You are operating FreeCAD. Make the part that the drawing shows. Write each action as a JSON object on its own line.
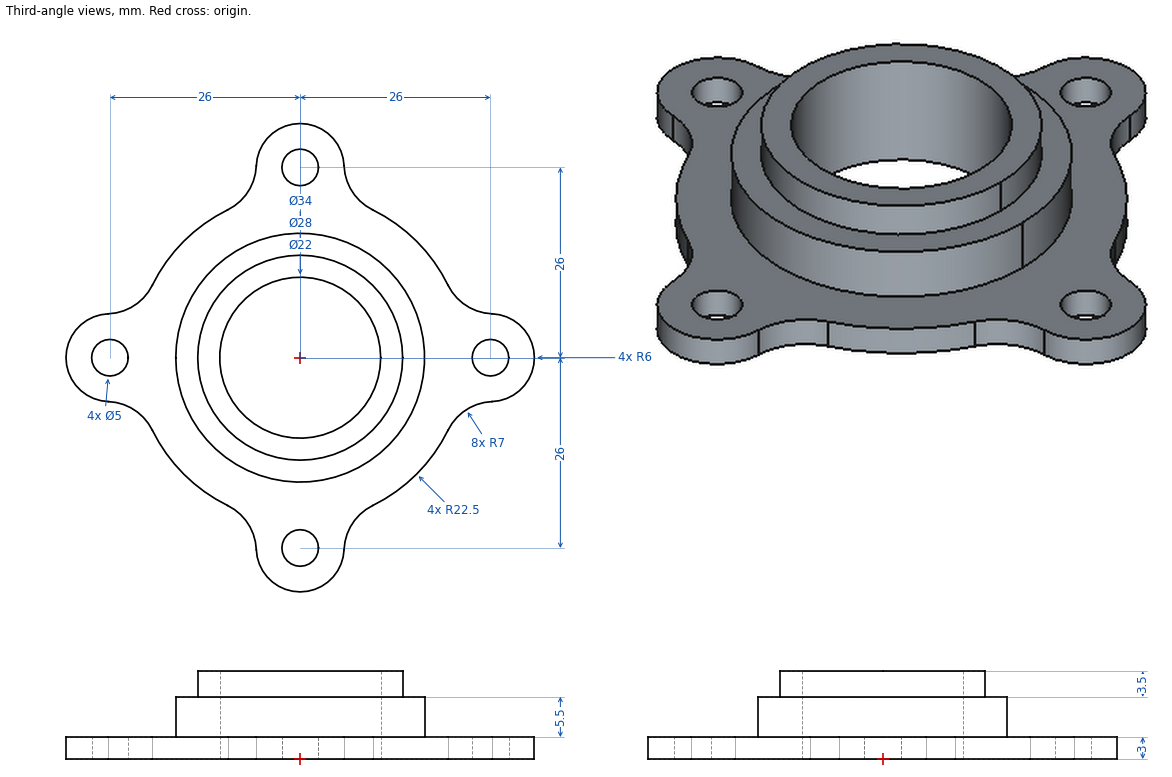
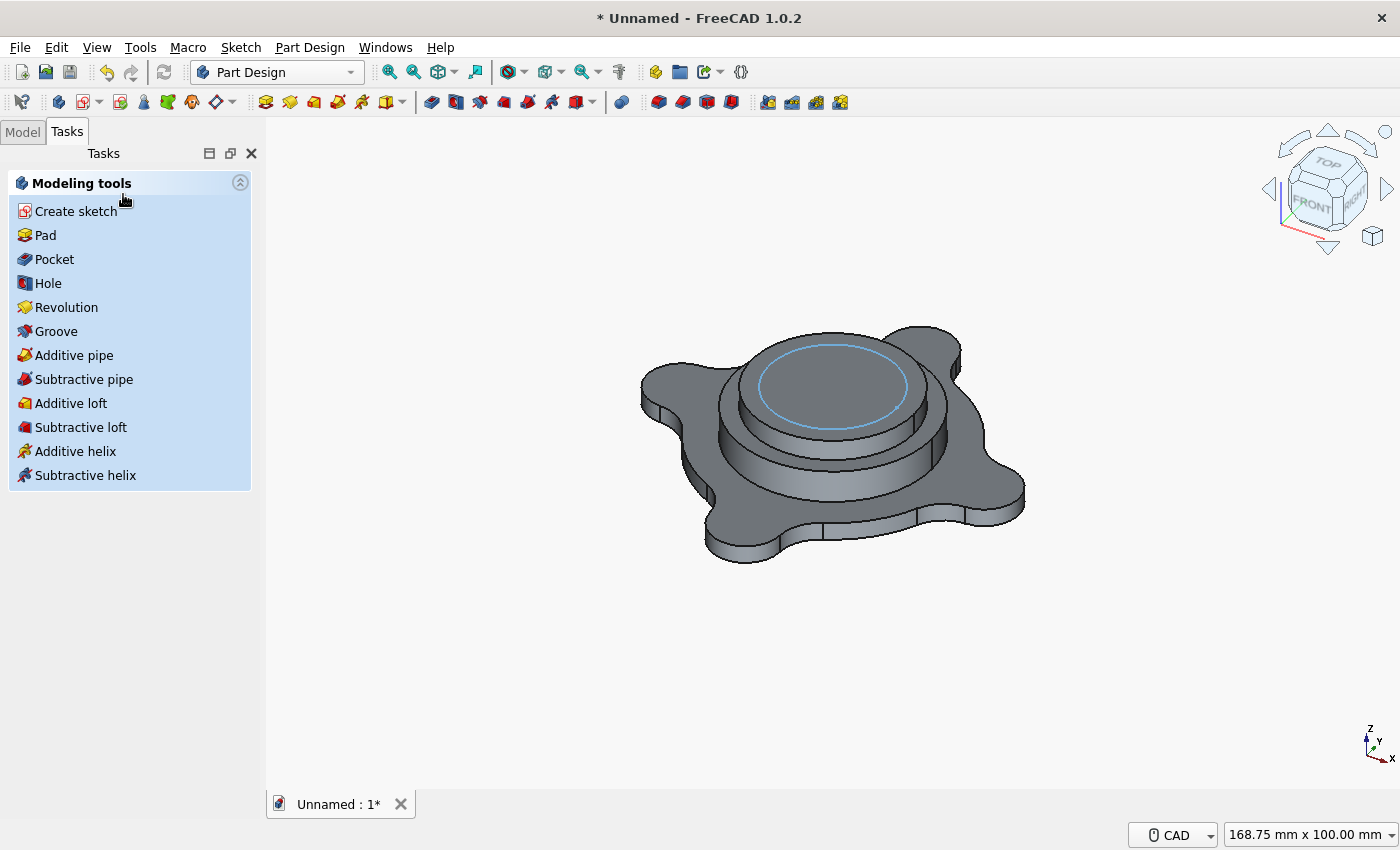
{"action": "left_click", "coordinate": [432, 102]}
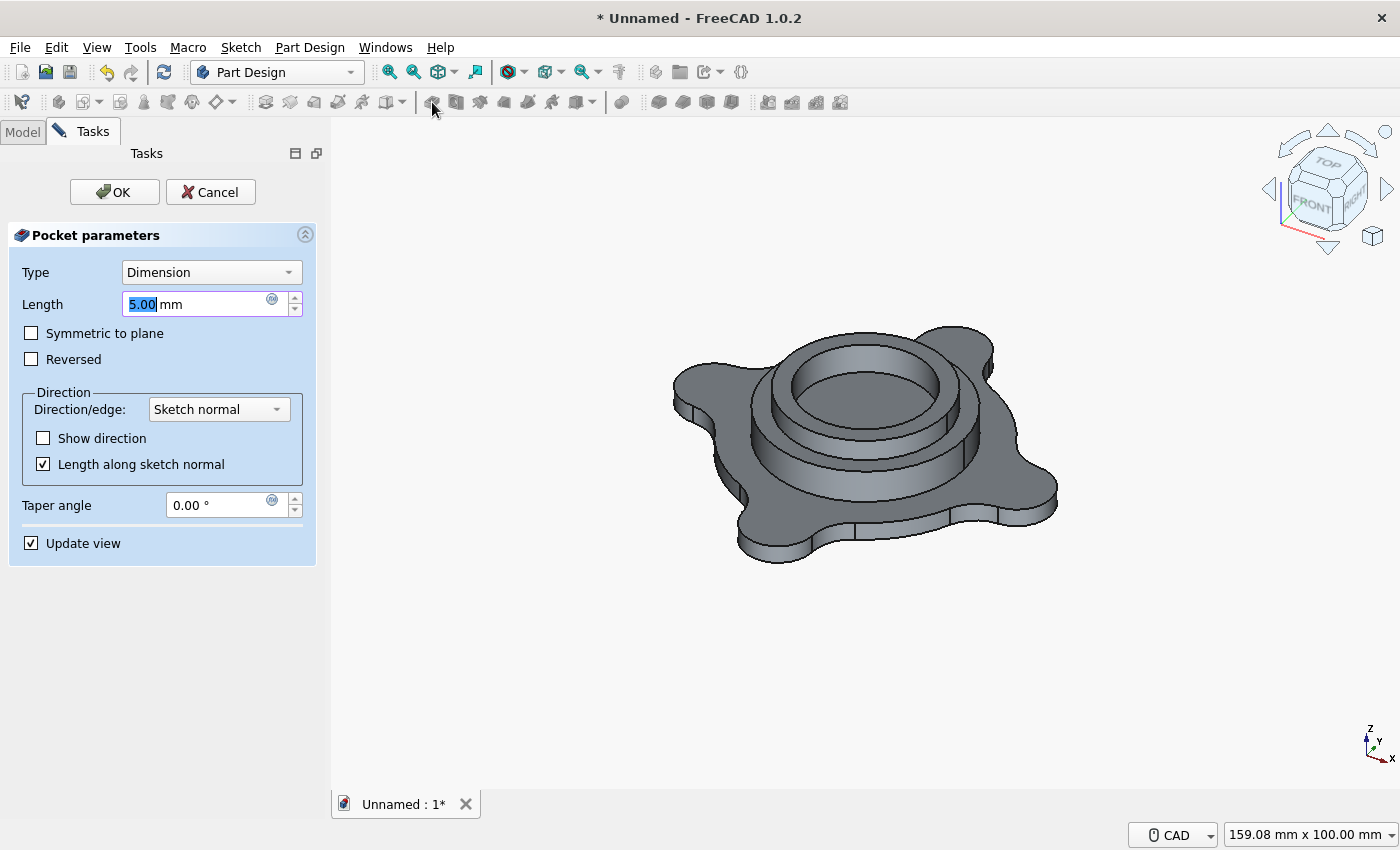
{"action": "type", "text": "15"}
{"action": "key", "text": "Tab"}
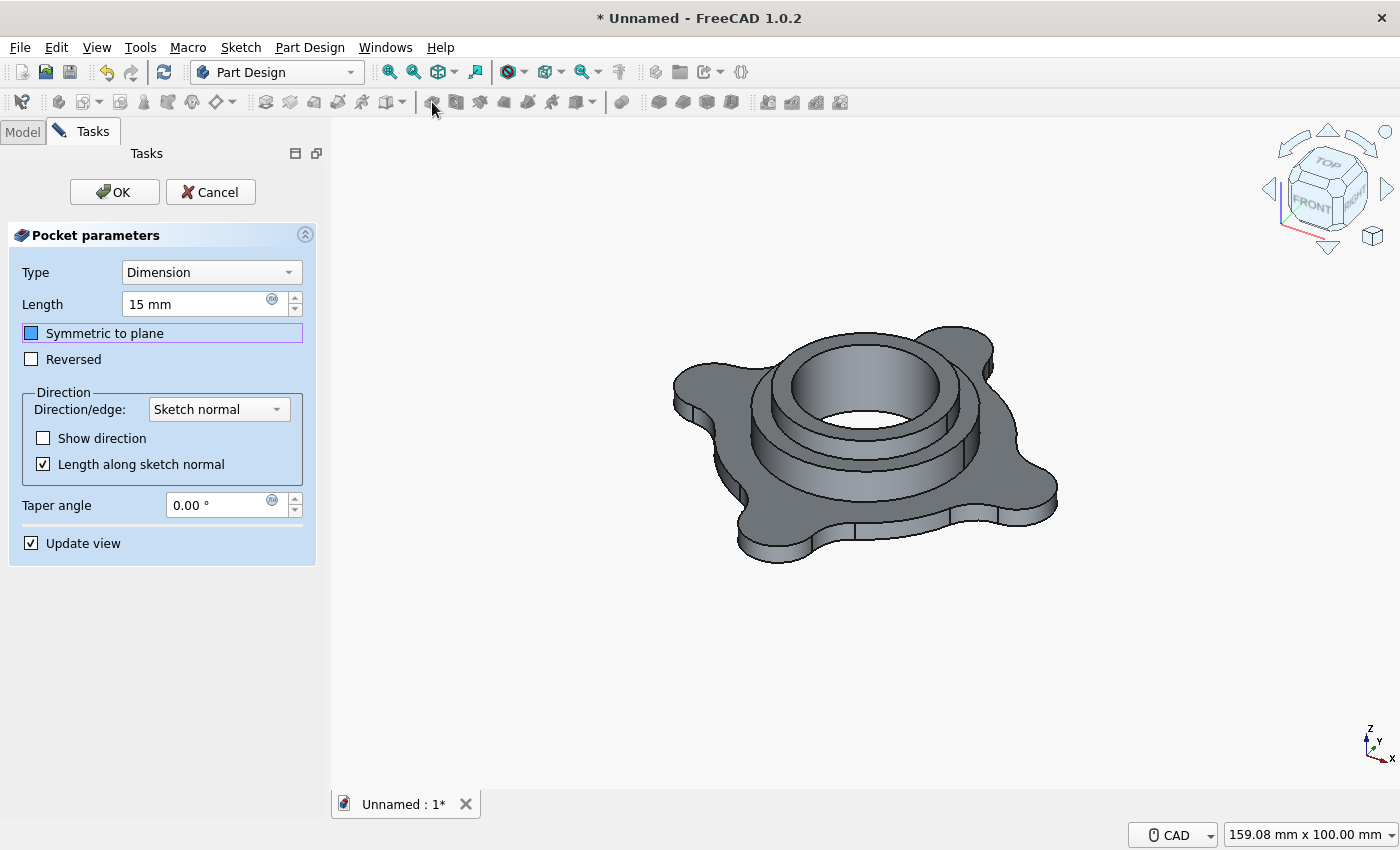
{"action": "left_click", "coordinate": [115, 192]}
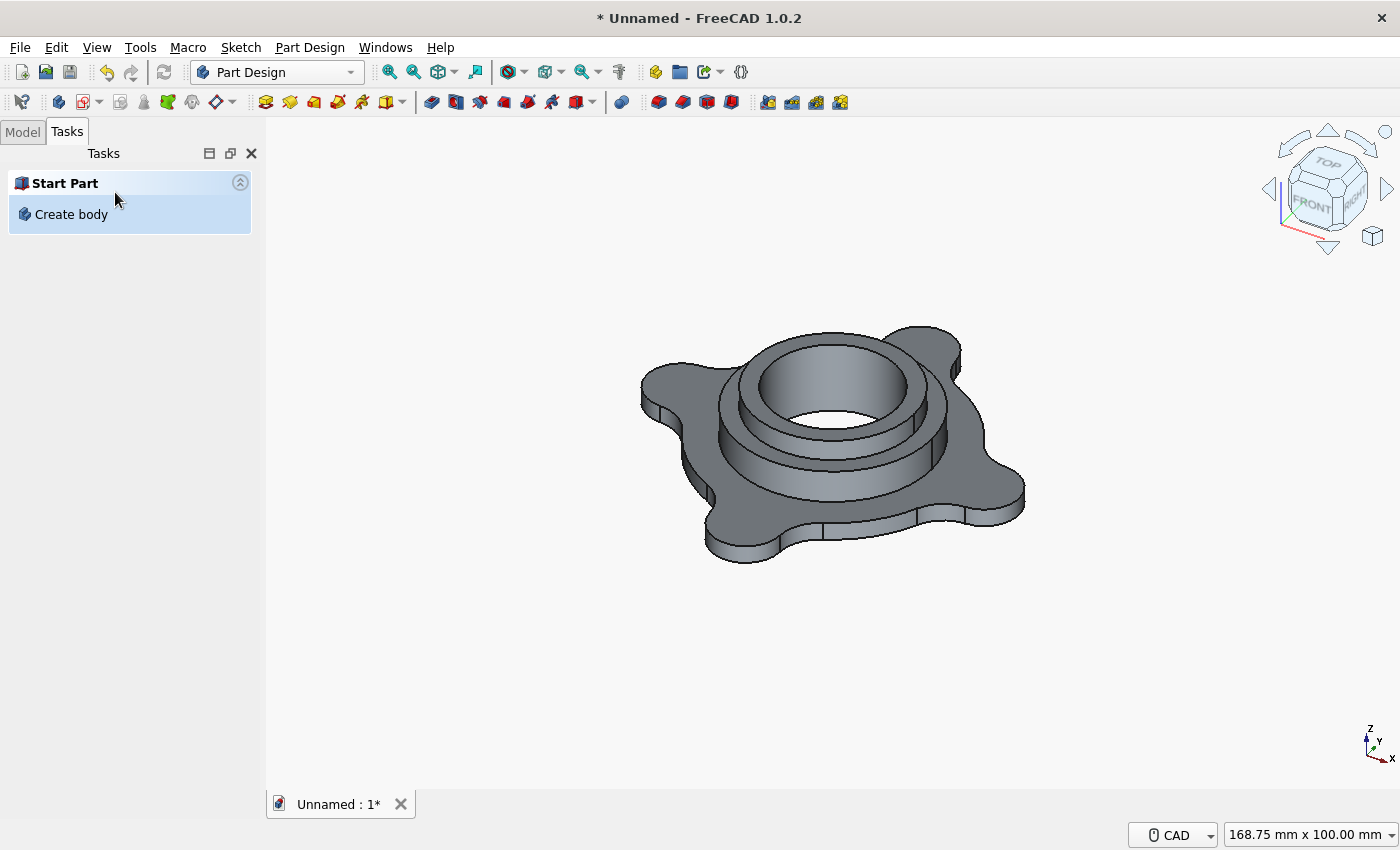
{"action": "left_click", "coordinate": [741, 527]}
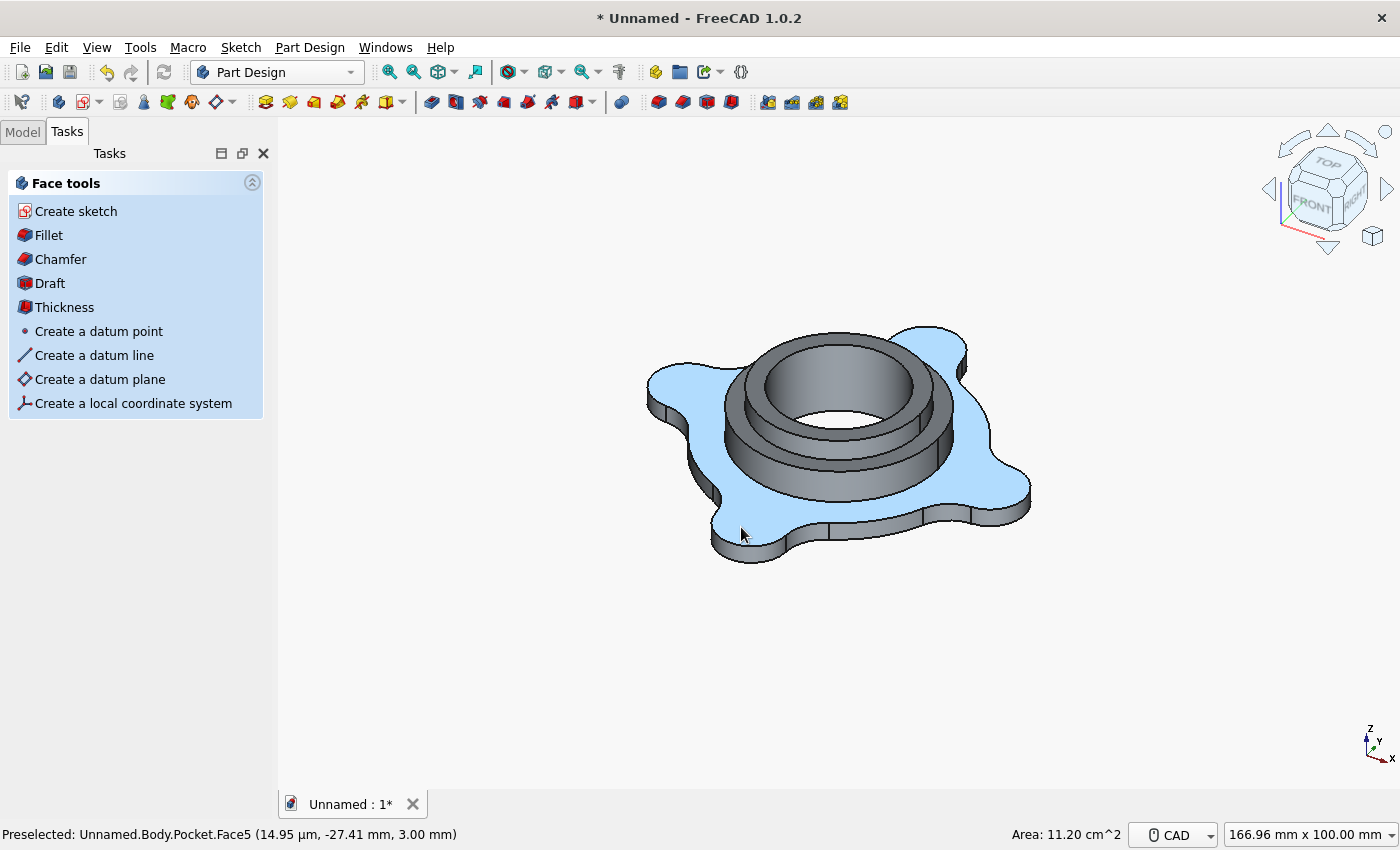
{"action": "left_click", "coordinate": [84, 102]}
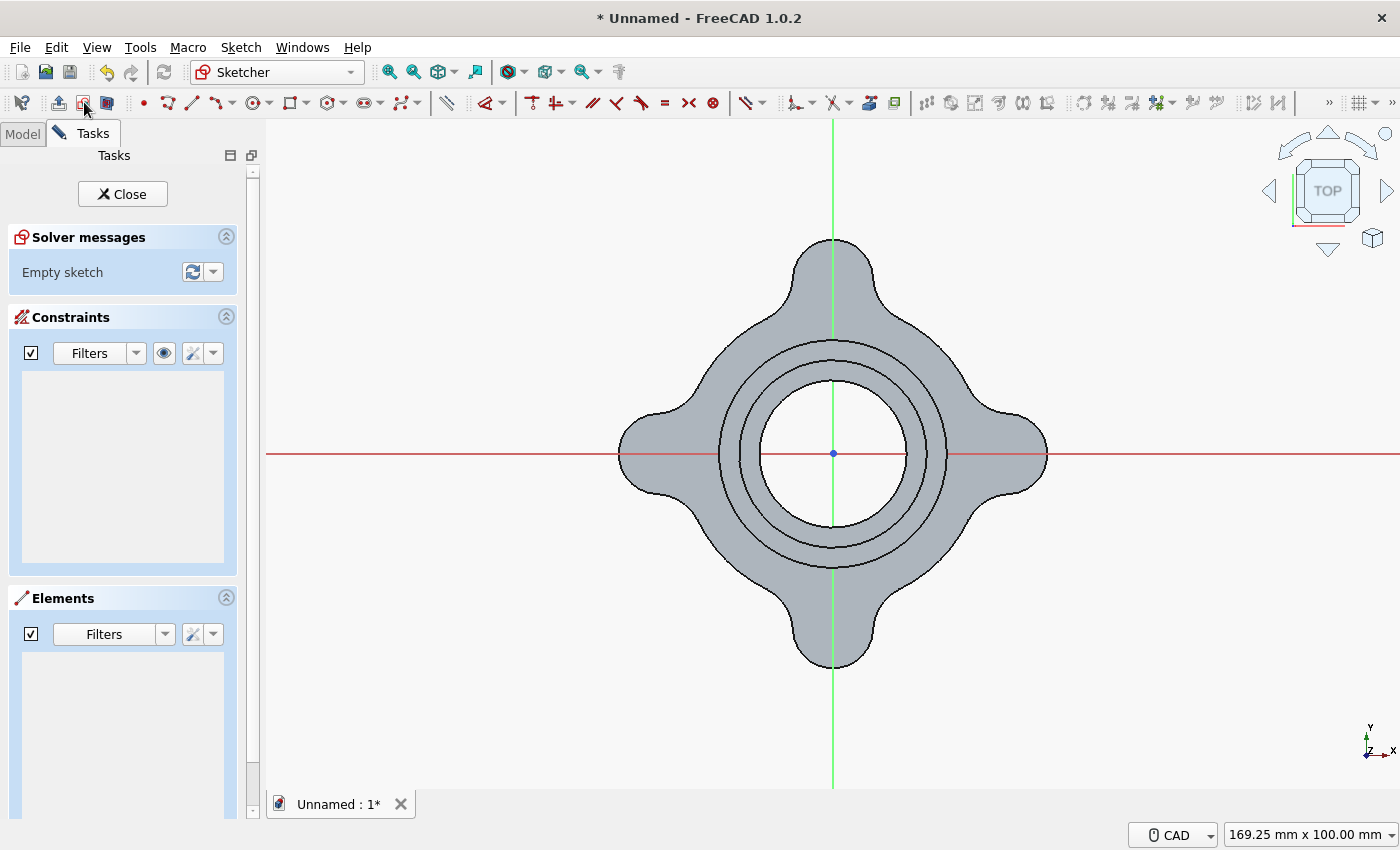
{"action": "left_click", "coordinate": [108, 104]}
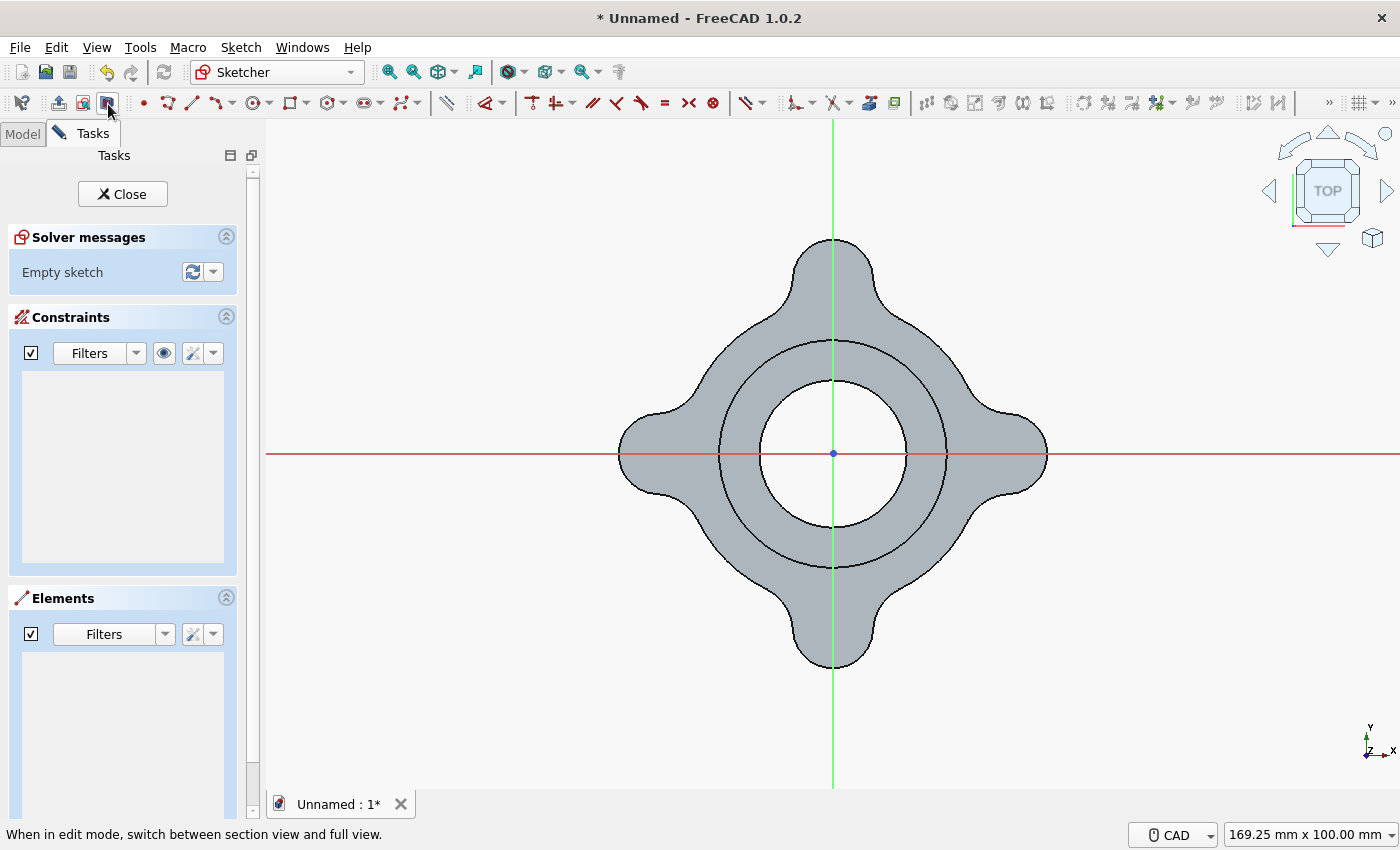
{"action": "left_click", "coordinate": [254, 104]}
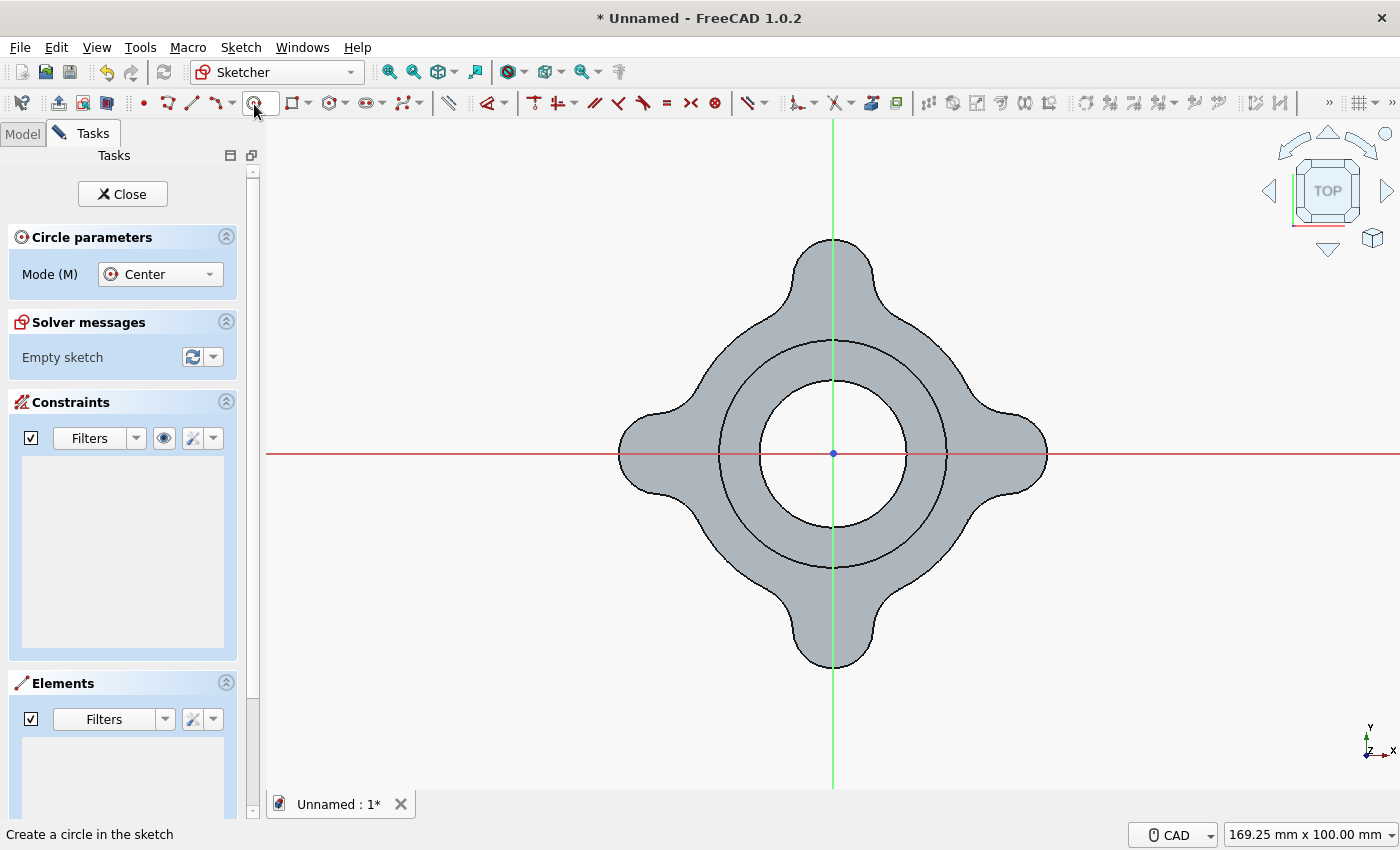
{"action": "scroll", "coordinate": [659, 454], "scroll_direction": "up", "scroll_amount": 2}